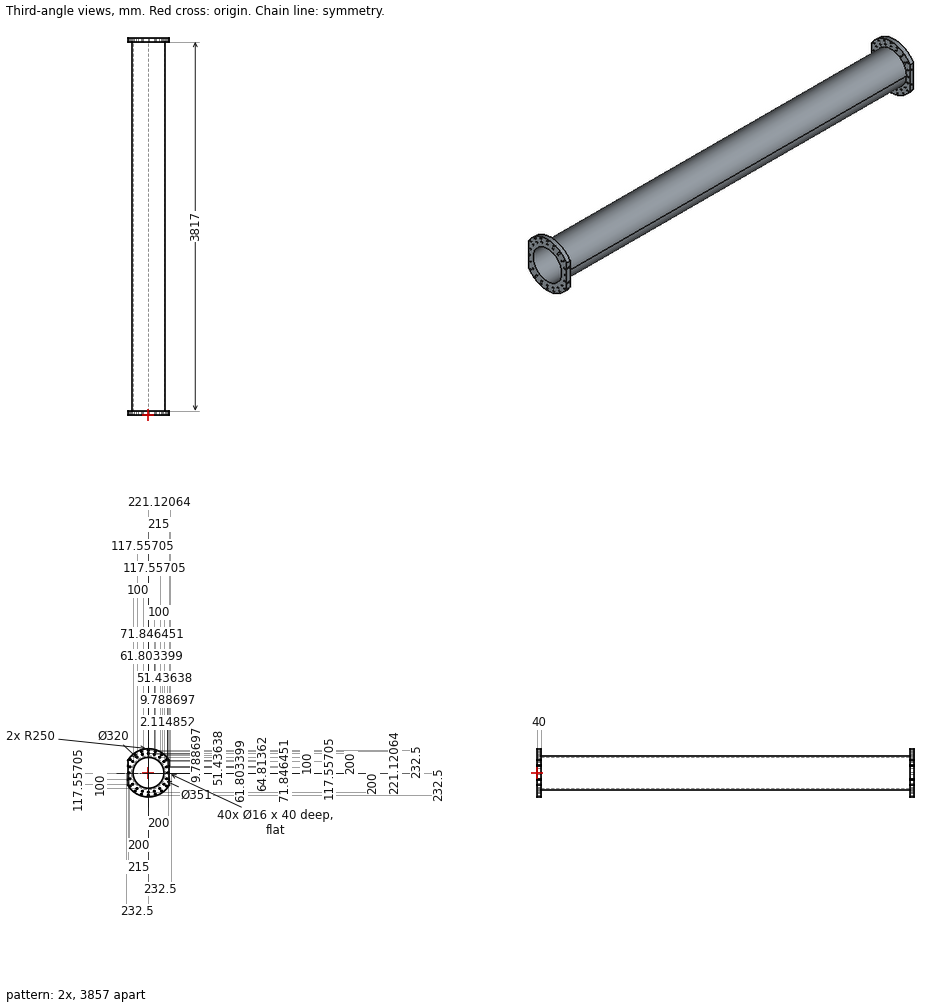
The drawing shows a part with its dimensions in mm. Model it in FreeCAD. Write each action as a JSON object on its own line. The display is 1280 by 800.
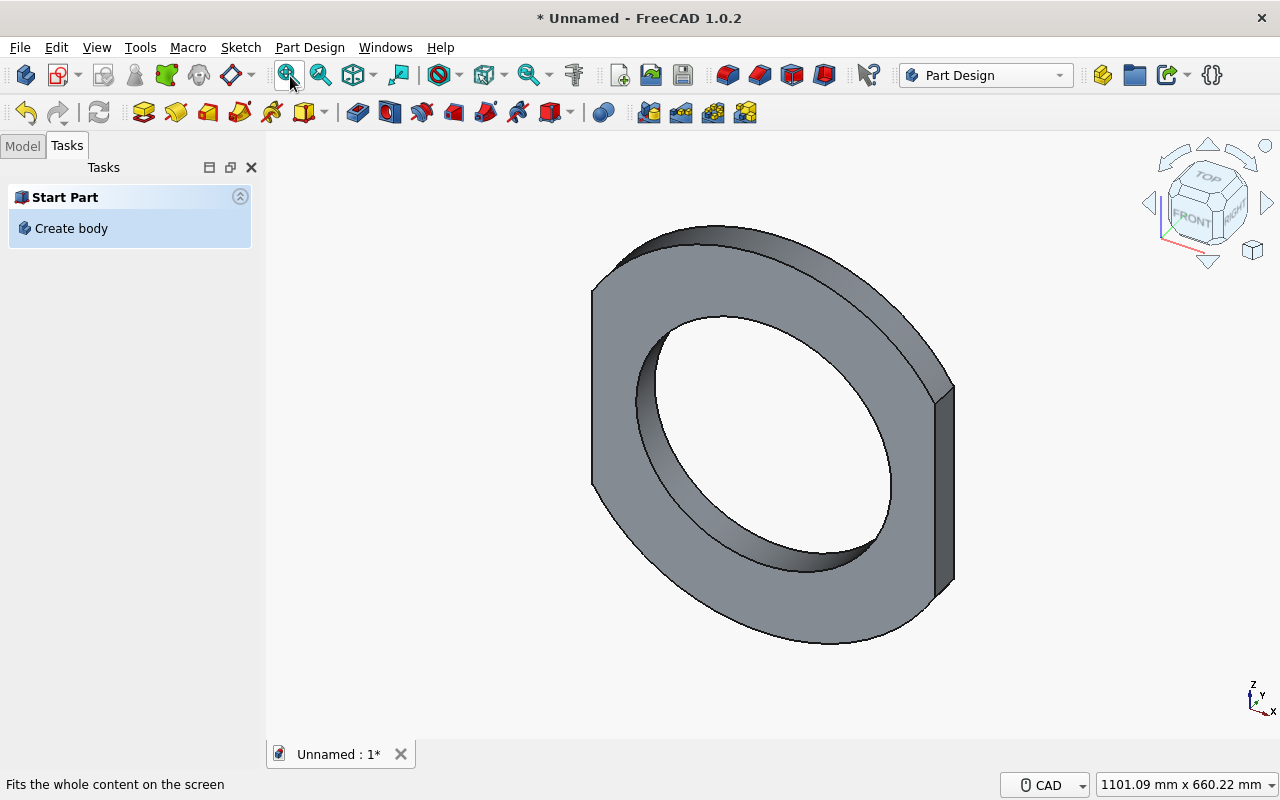
{"action": "key", "text": "4"}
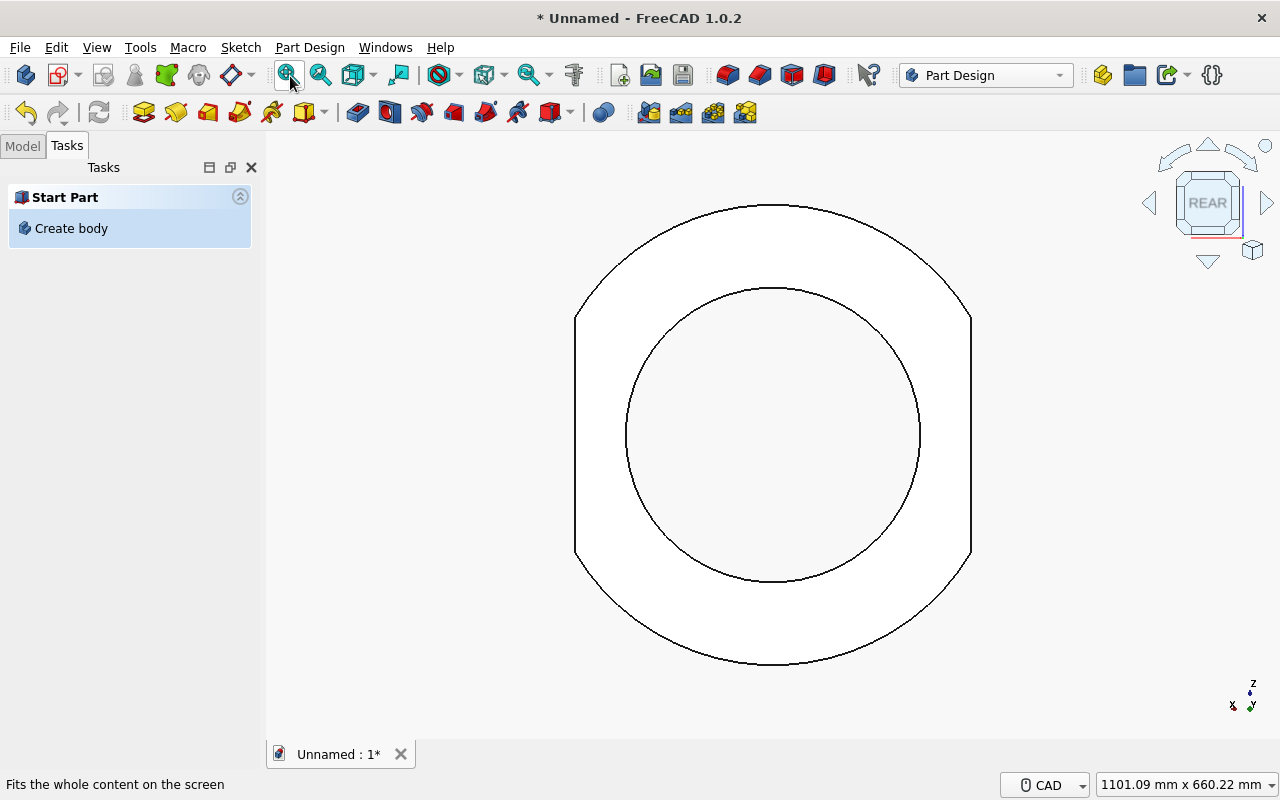
{"action": "left_click", "coordinate": [773, 237]}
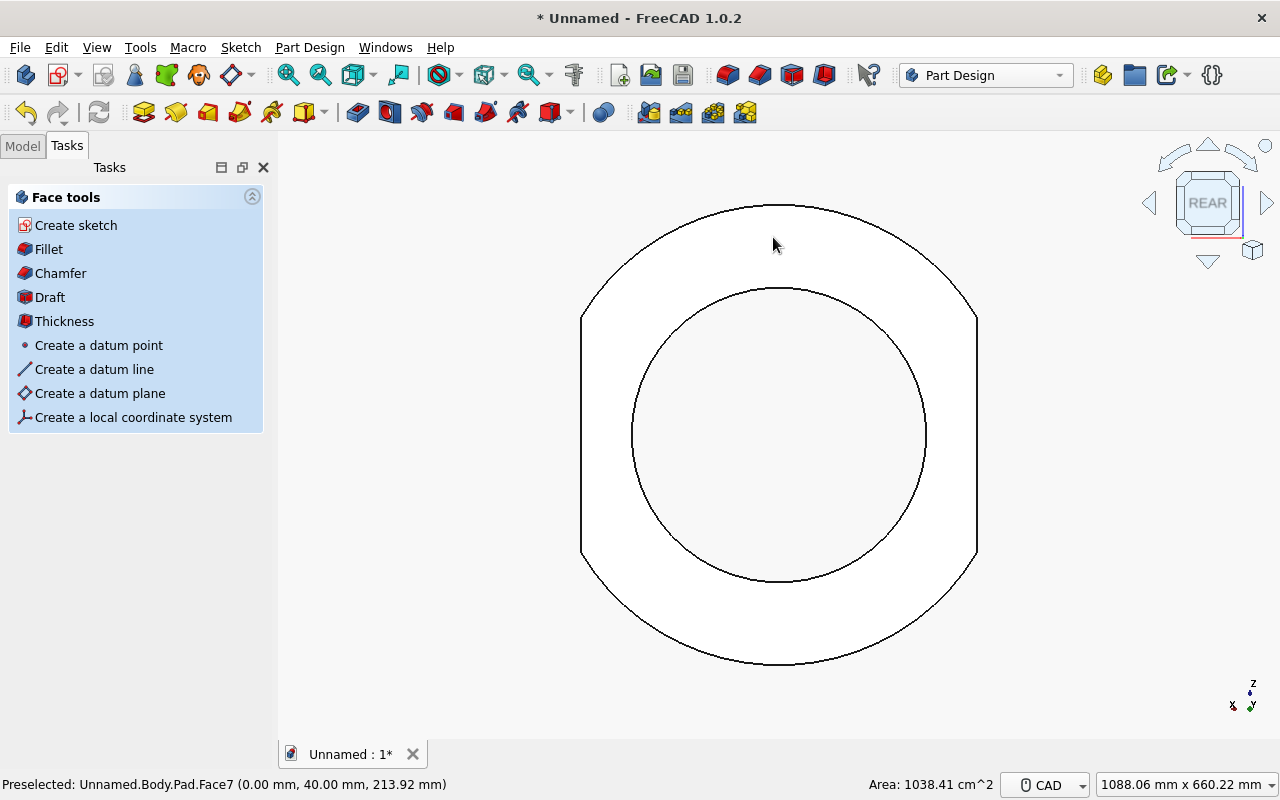
{"action": "left_click", "coordinate": [58, 76]}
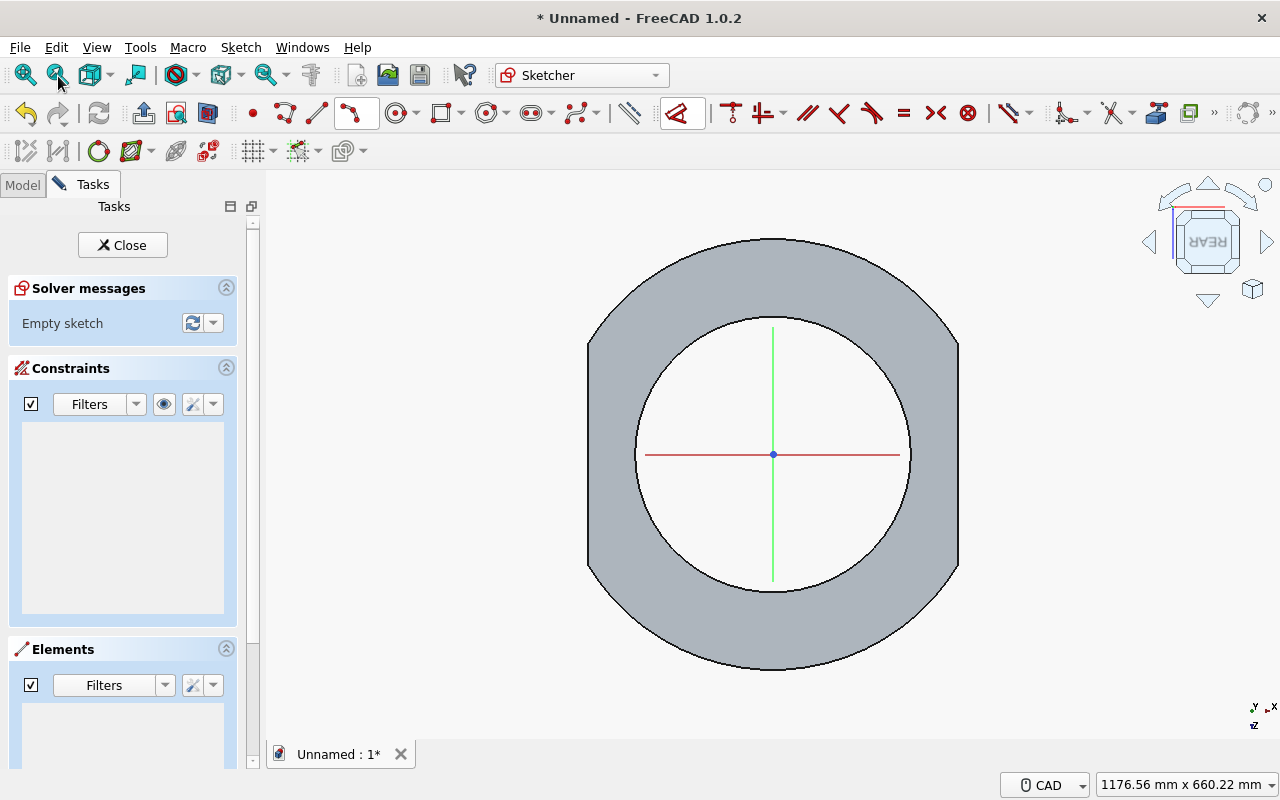
{"action": "key", "text": "g c"}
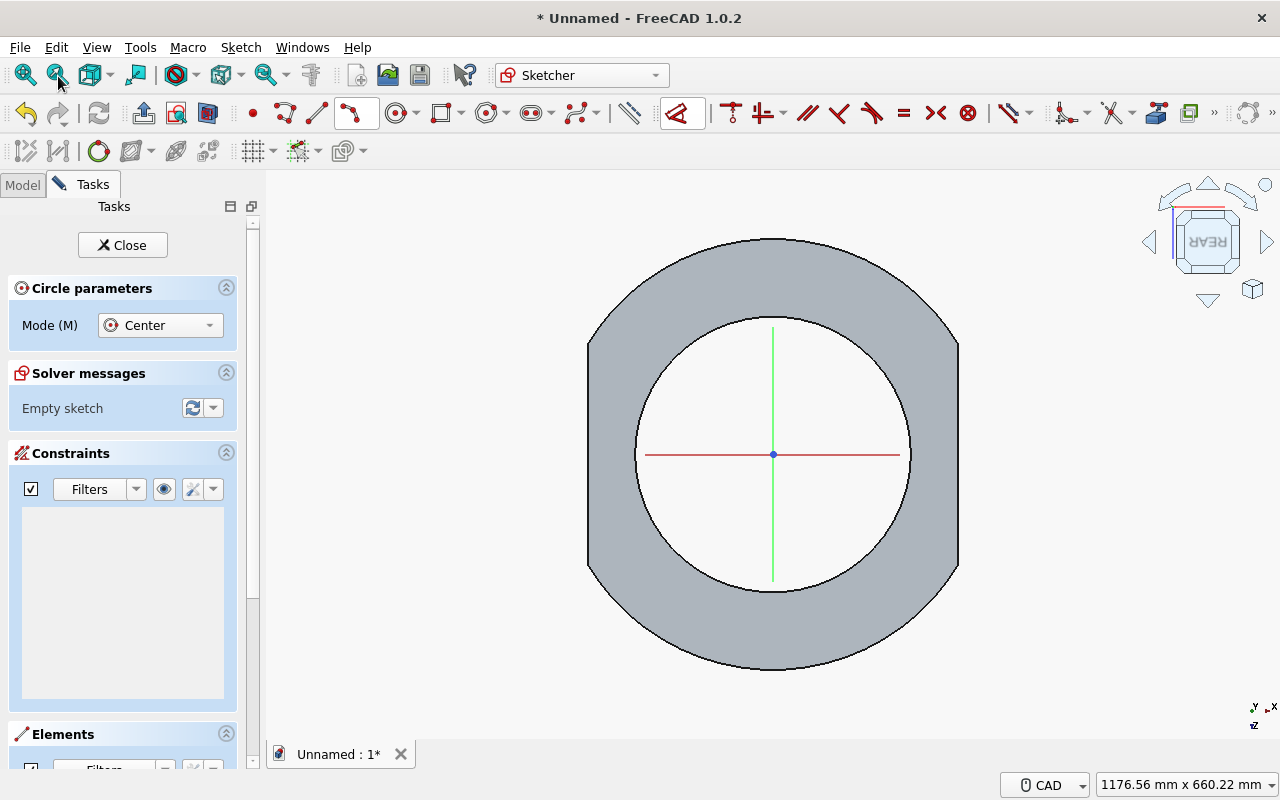
{"action": "left_click", "coordinate": [773, 454]}
{"action": "mouse_move", "coordinate": [880, 348]}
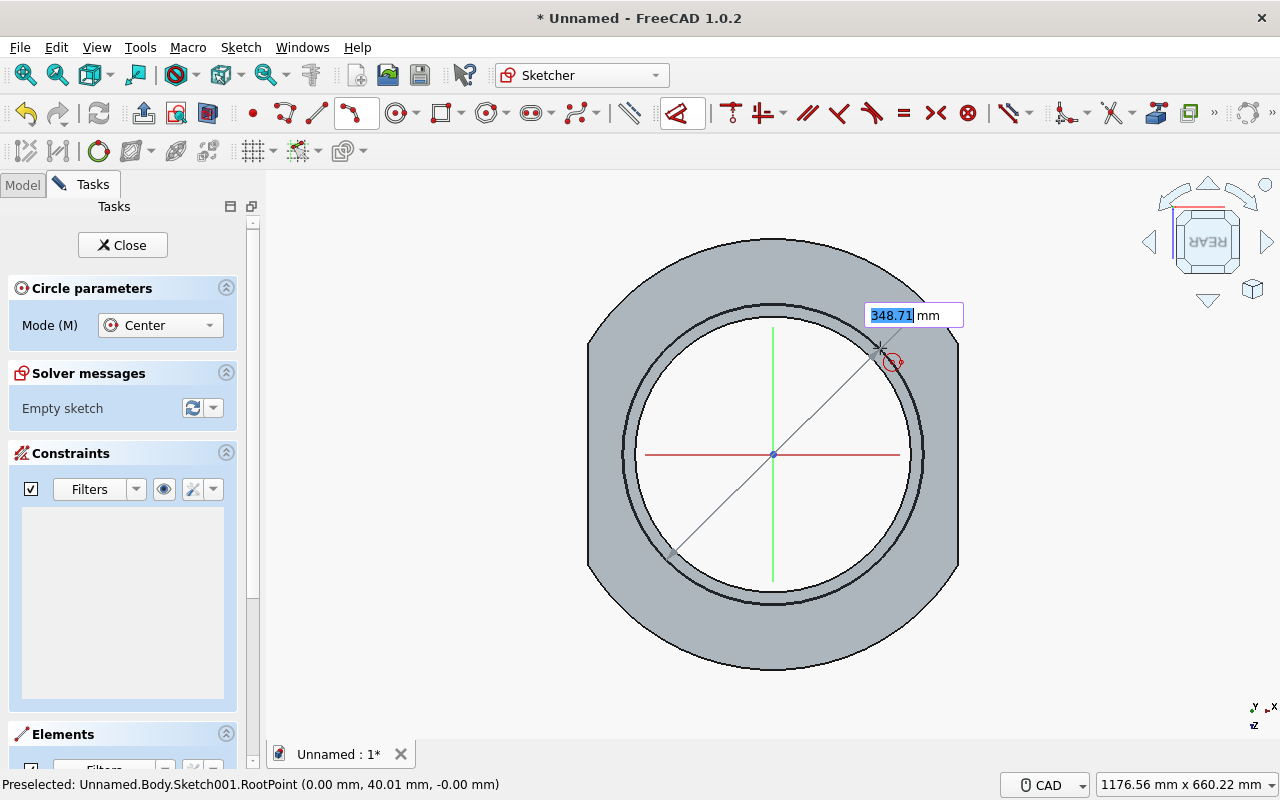
{"action": "type", "text": "351"}
{"action": "key", "text": "Return"}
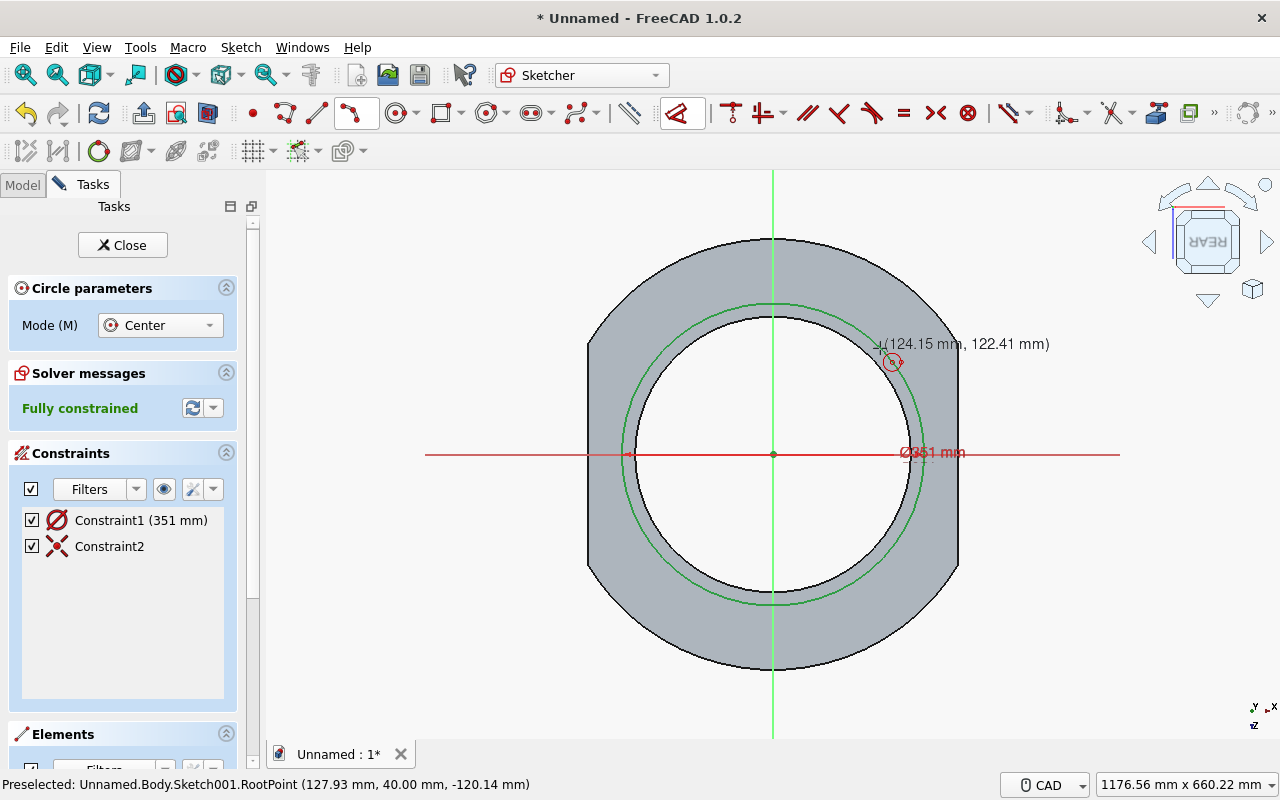
{"action": "left_click", "coordinate": [773, 454]}
{"action": "mouse_move", "coordinate": [871, 357]}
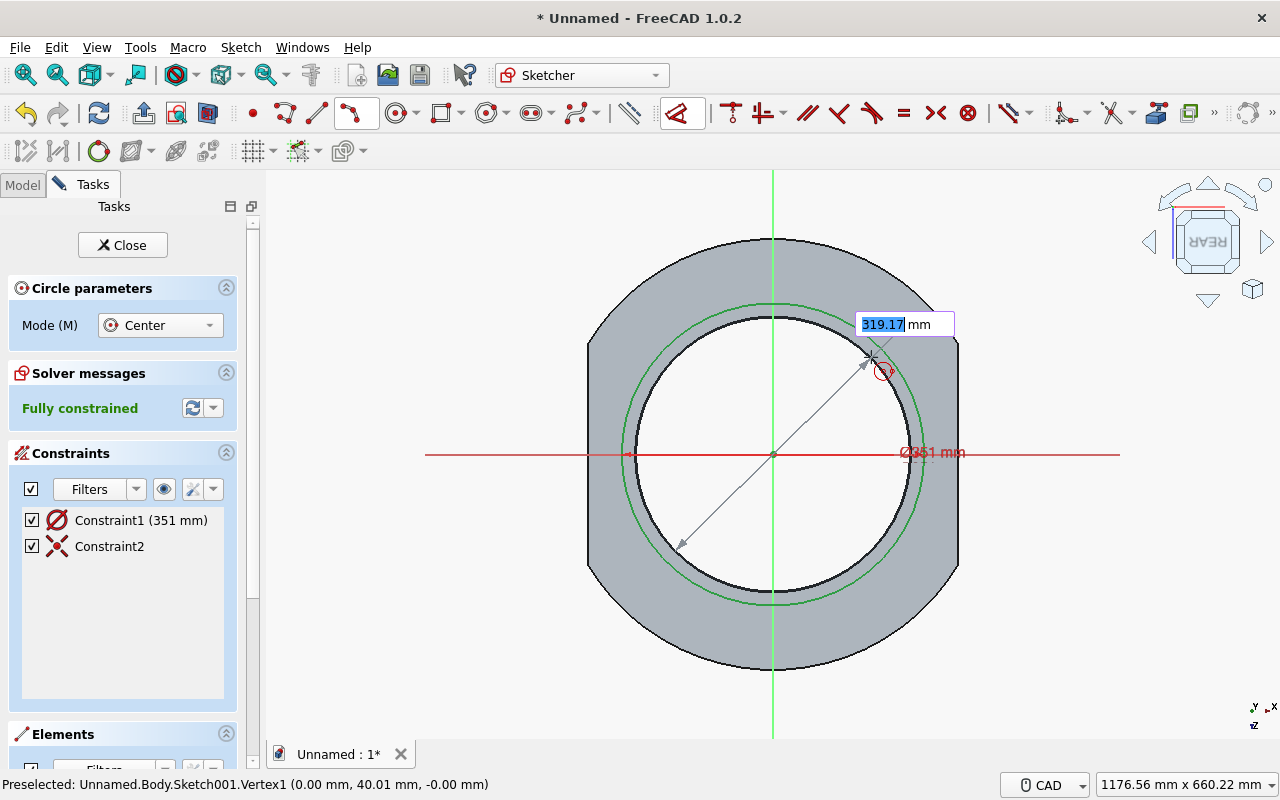
{"action": "type", "text": "320"}
{"action": "key", "text": "Return"}
{"action": "key", "text": "Escape"}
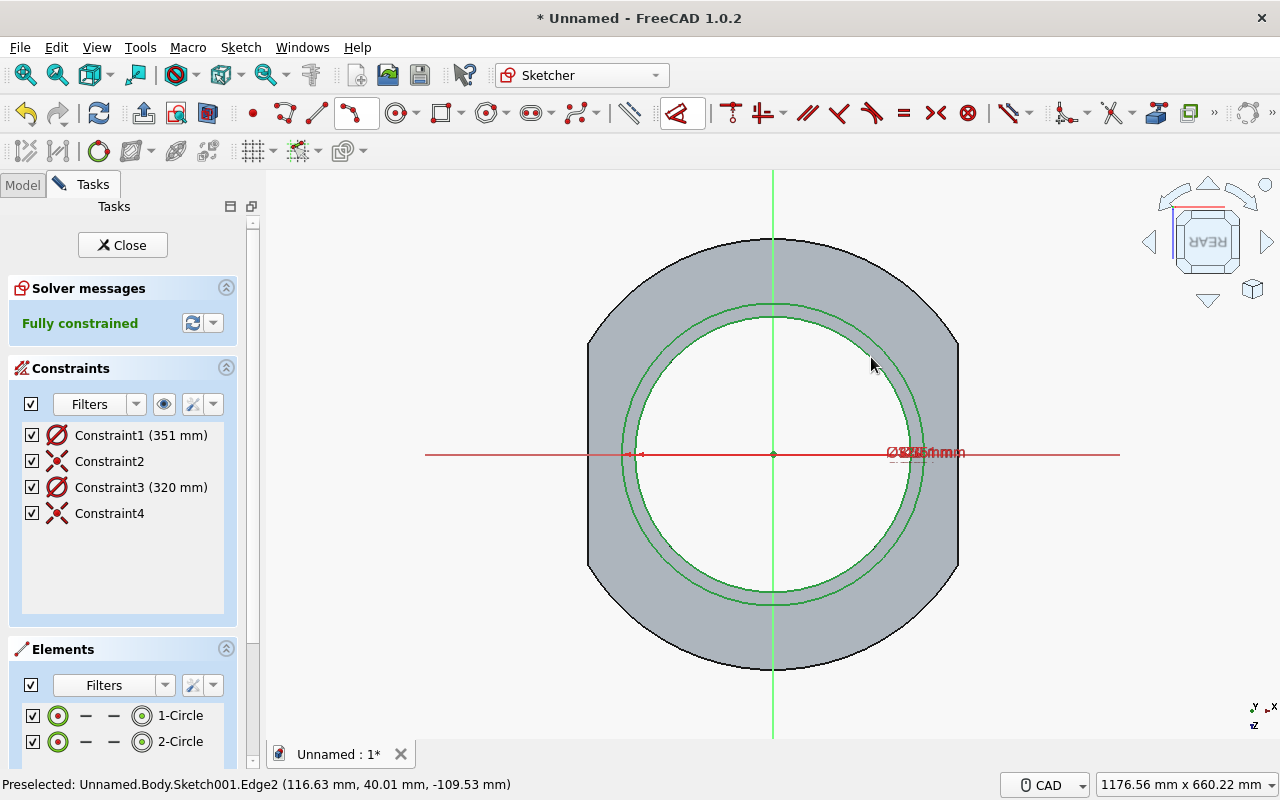
{"action": "left_click", "coordinate": [123, 245]}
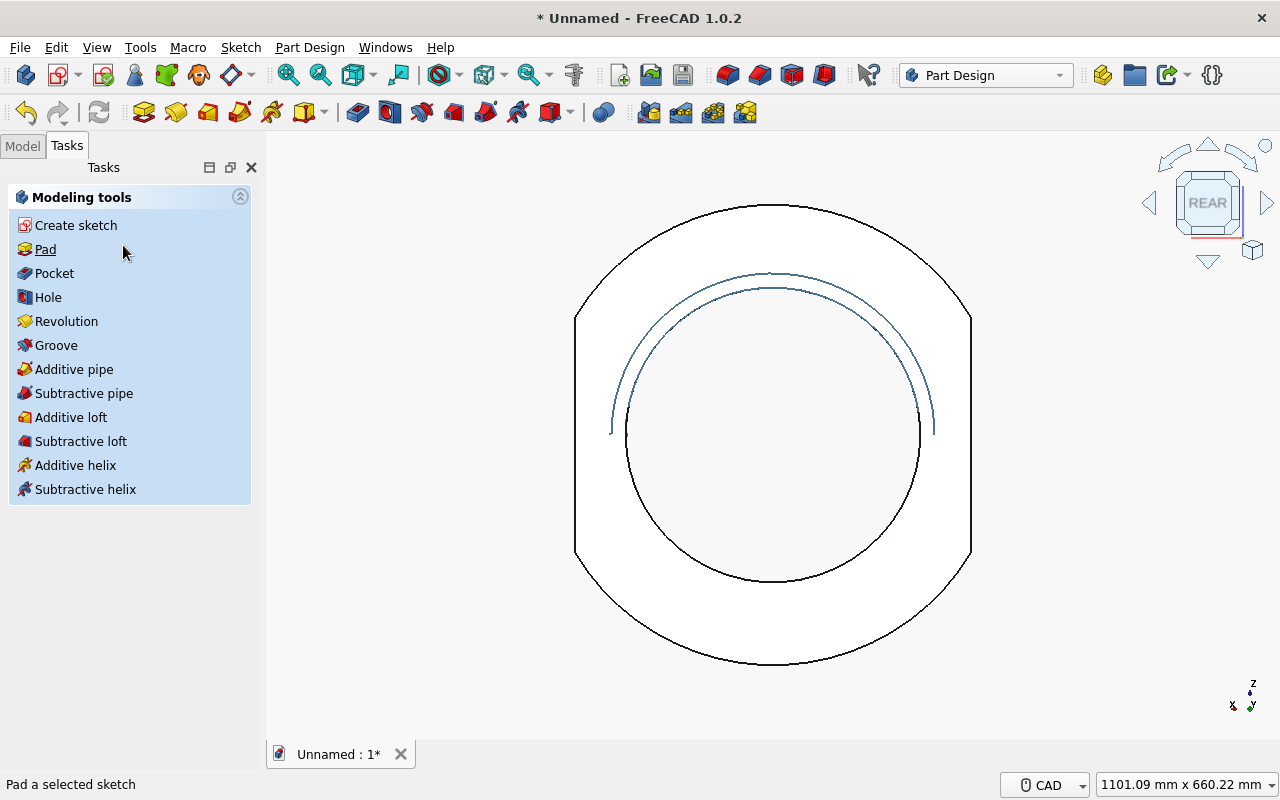
{"action": "left_click", "coordinate": [144, 112]}